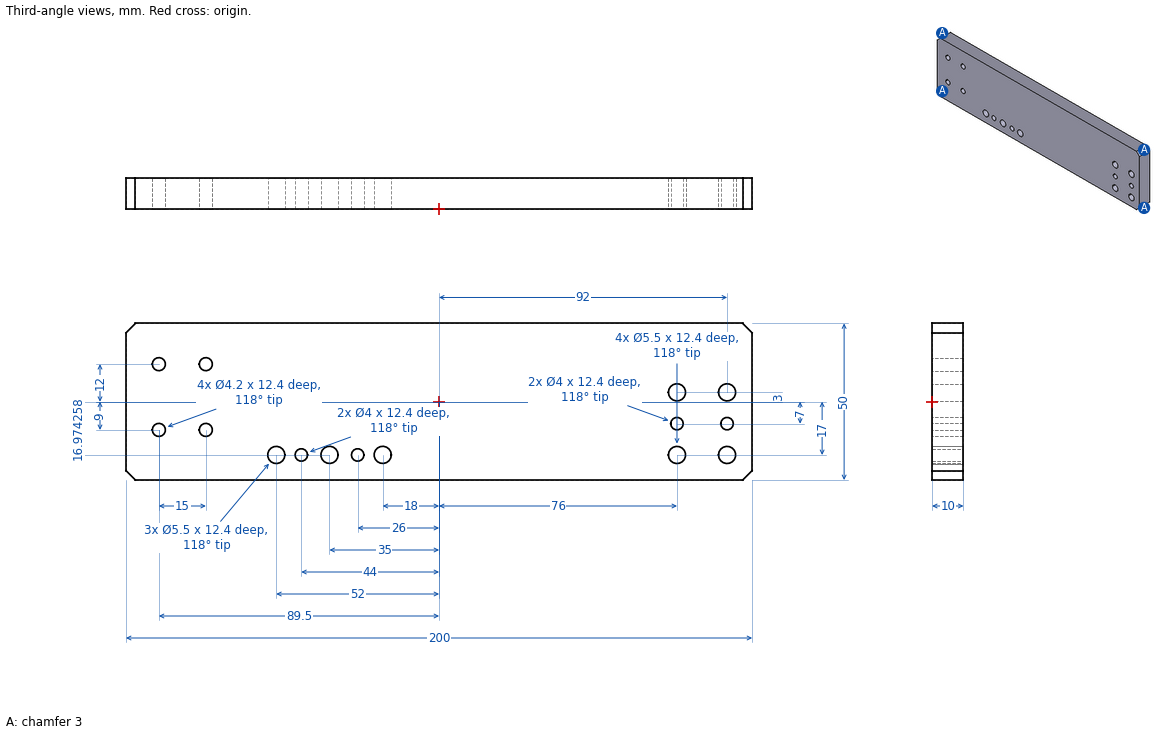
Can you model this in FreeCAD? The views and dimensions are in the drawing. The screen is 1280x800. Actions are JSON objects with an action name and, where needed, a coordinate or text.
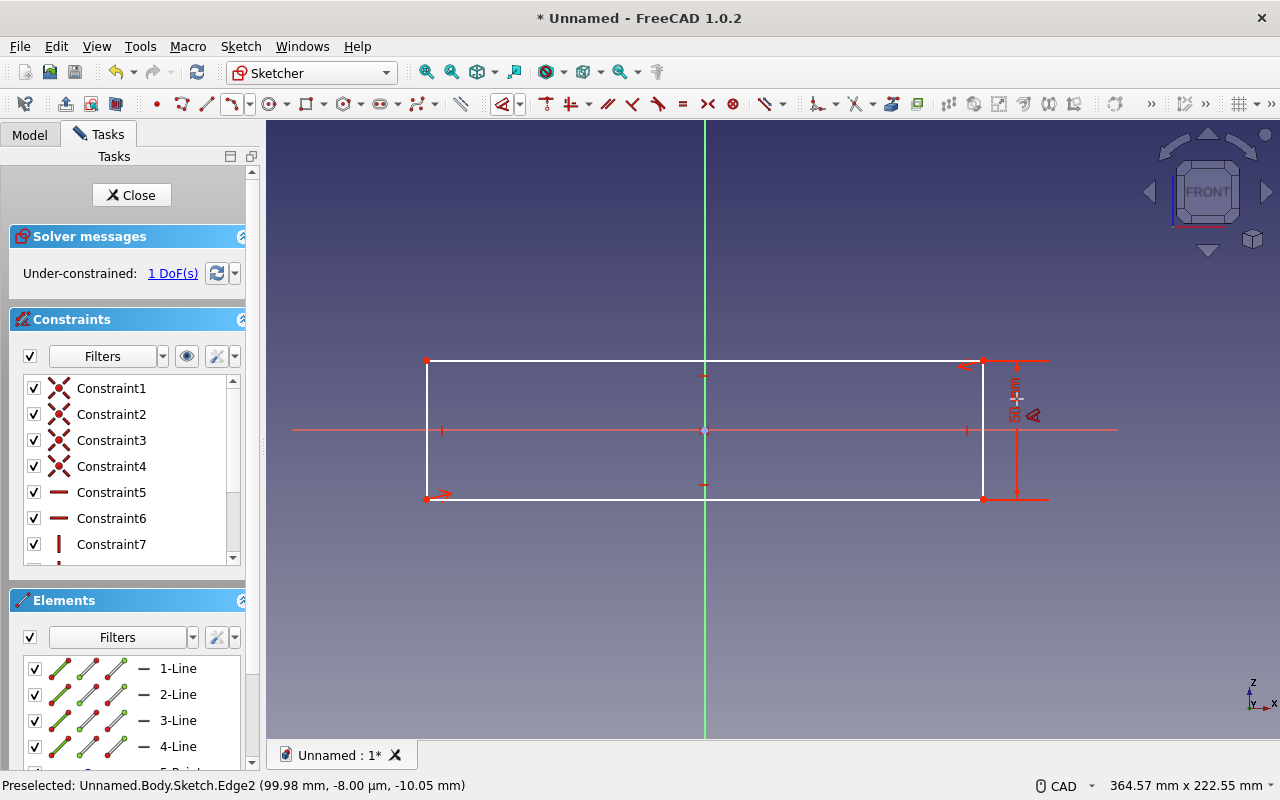
{"action": "left_click", "coordinate": [594, 500]}
{"action": "left_click", "coordinate": [577, 534]}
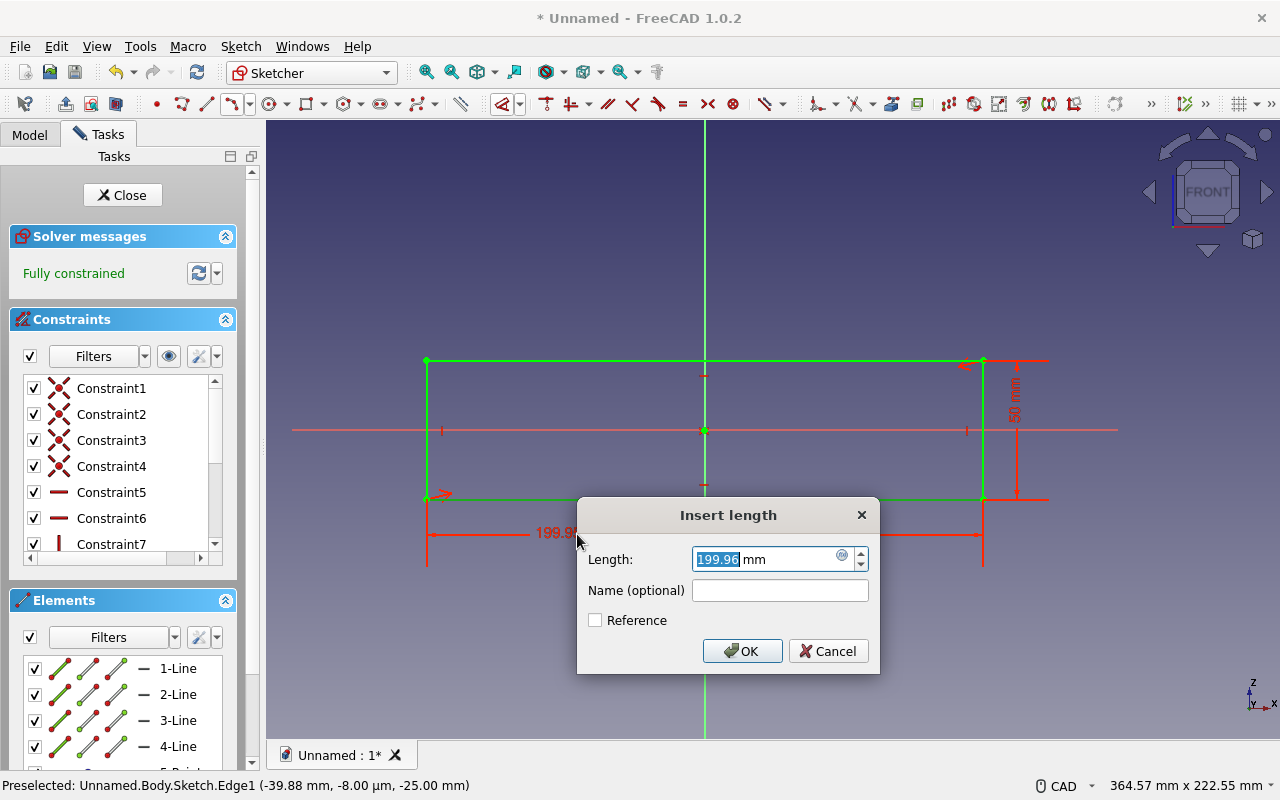
{"action": "type", "text": "200"}
{"action": "key", "text": "Return"}
{"action": "key", "text": "Escape"}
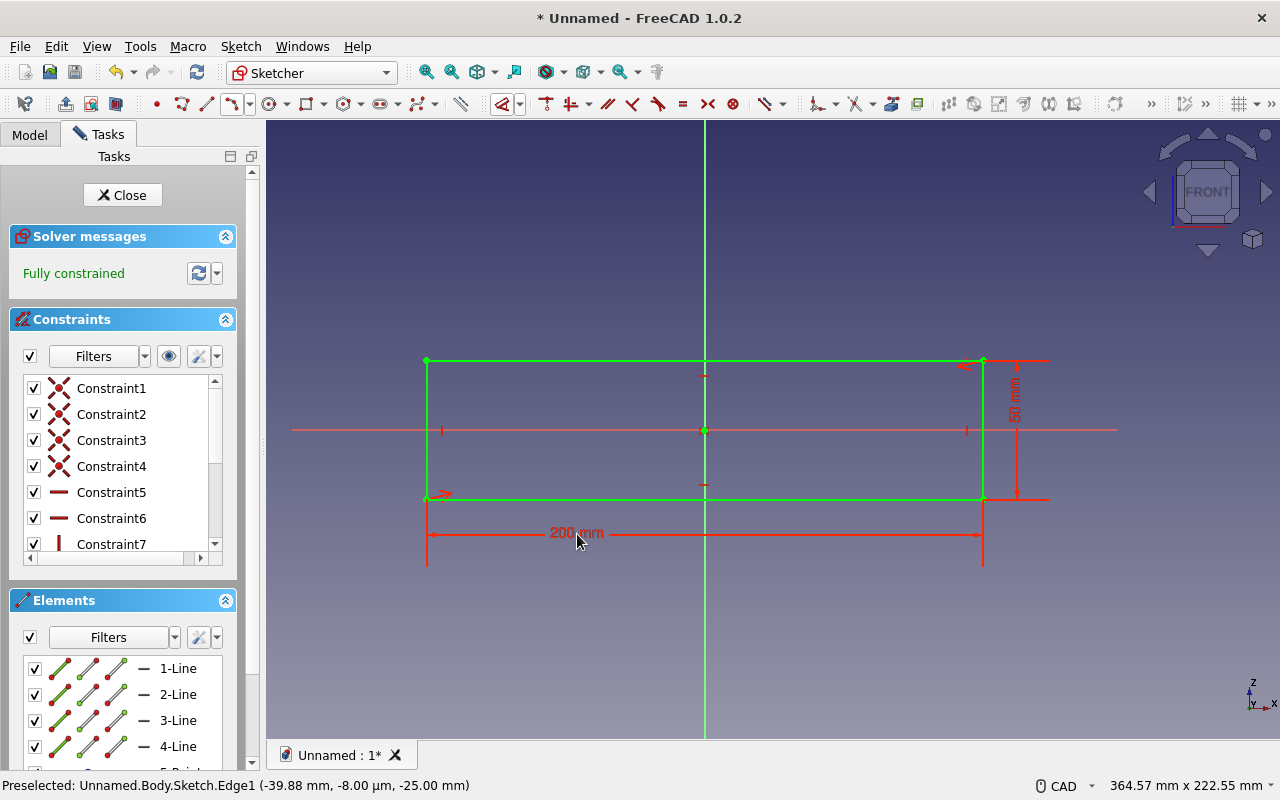
{"action": "left_click", "coordinate": [123, 195]}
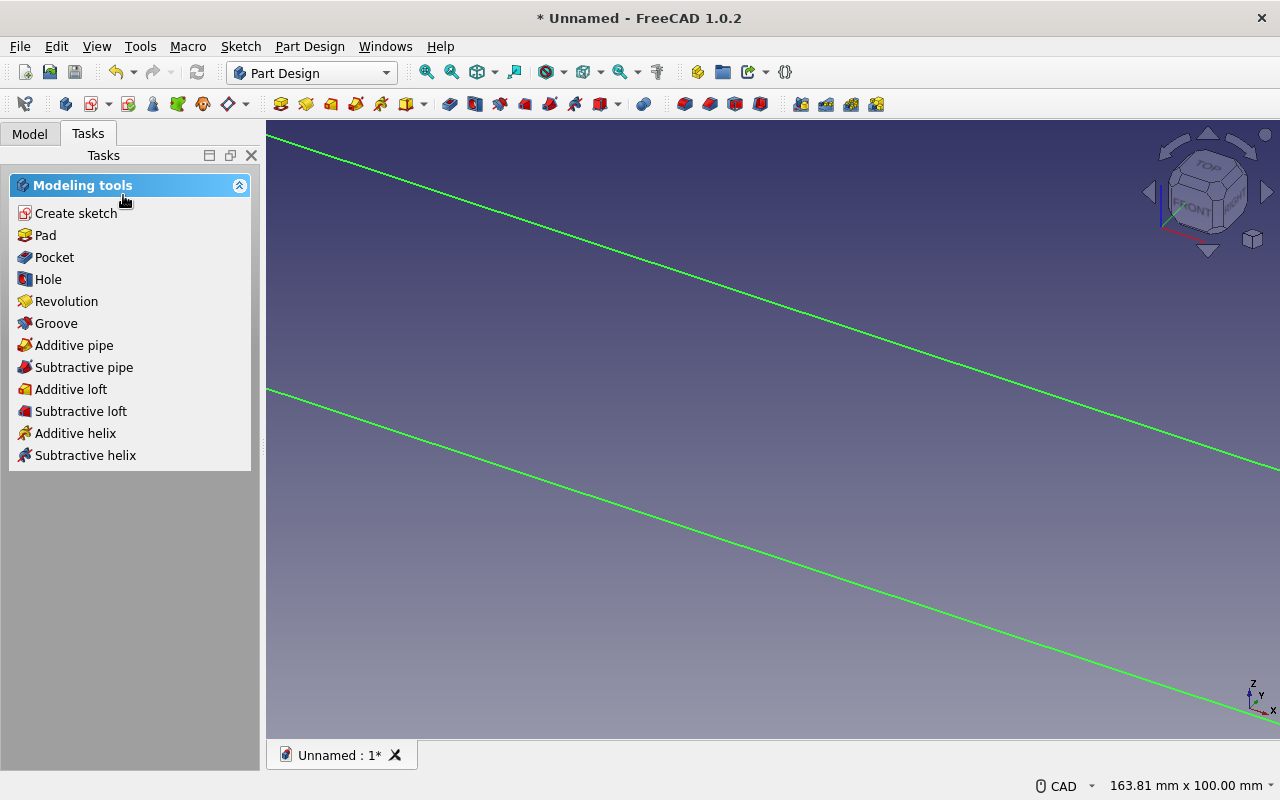
{"action": "left_click", "coordinate": [281, 104]}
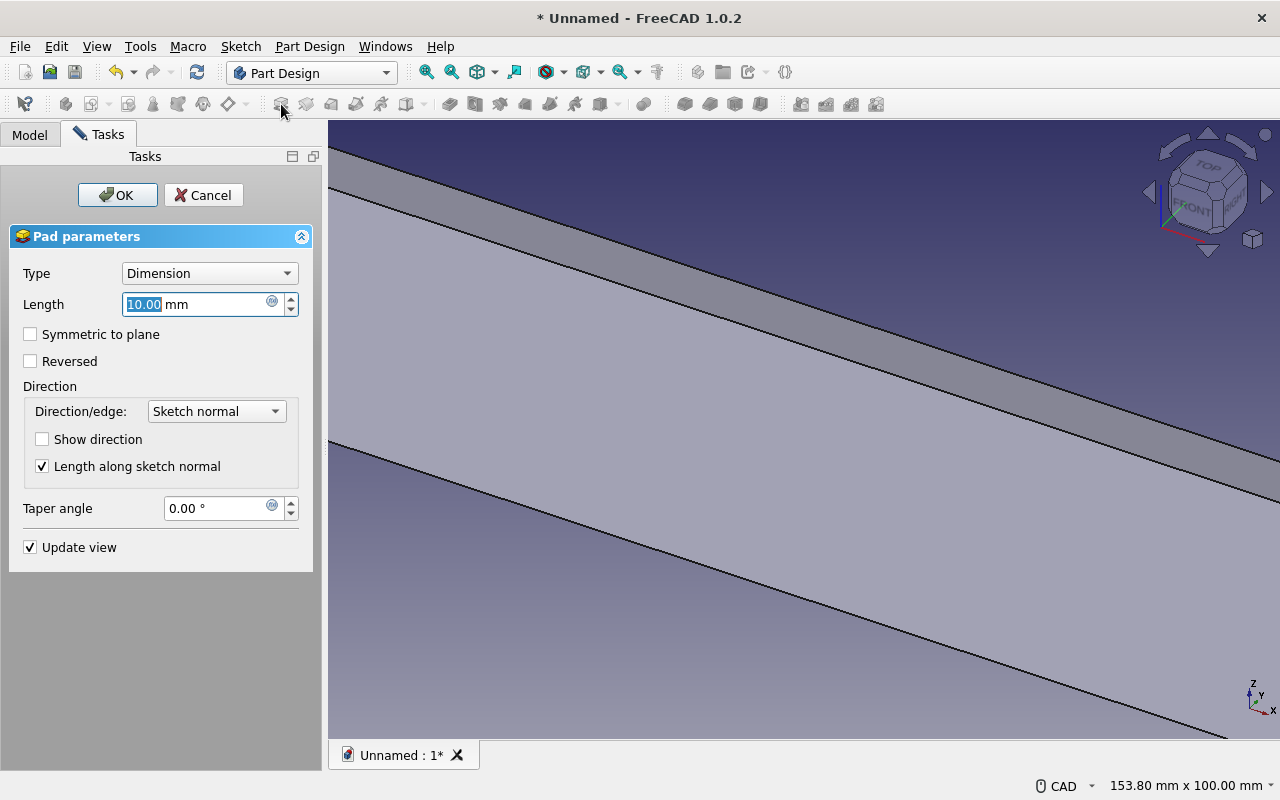
{"action": "type", "text": "10"}
{"action": "key", "text": "Tab"}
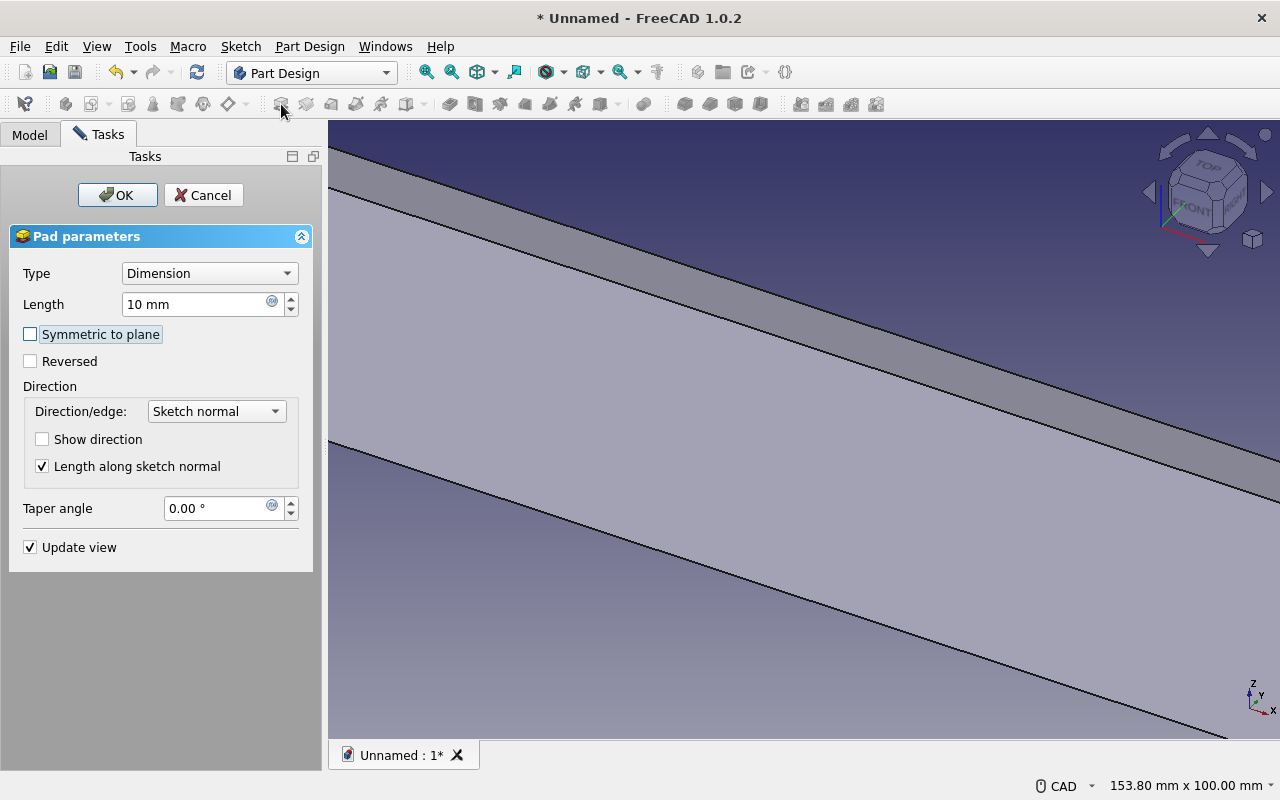
{"action": "left_click", "coordinate": [31, 361]}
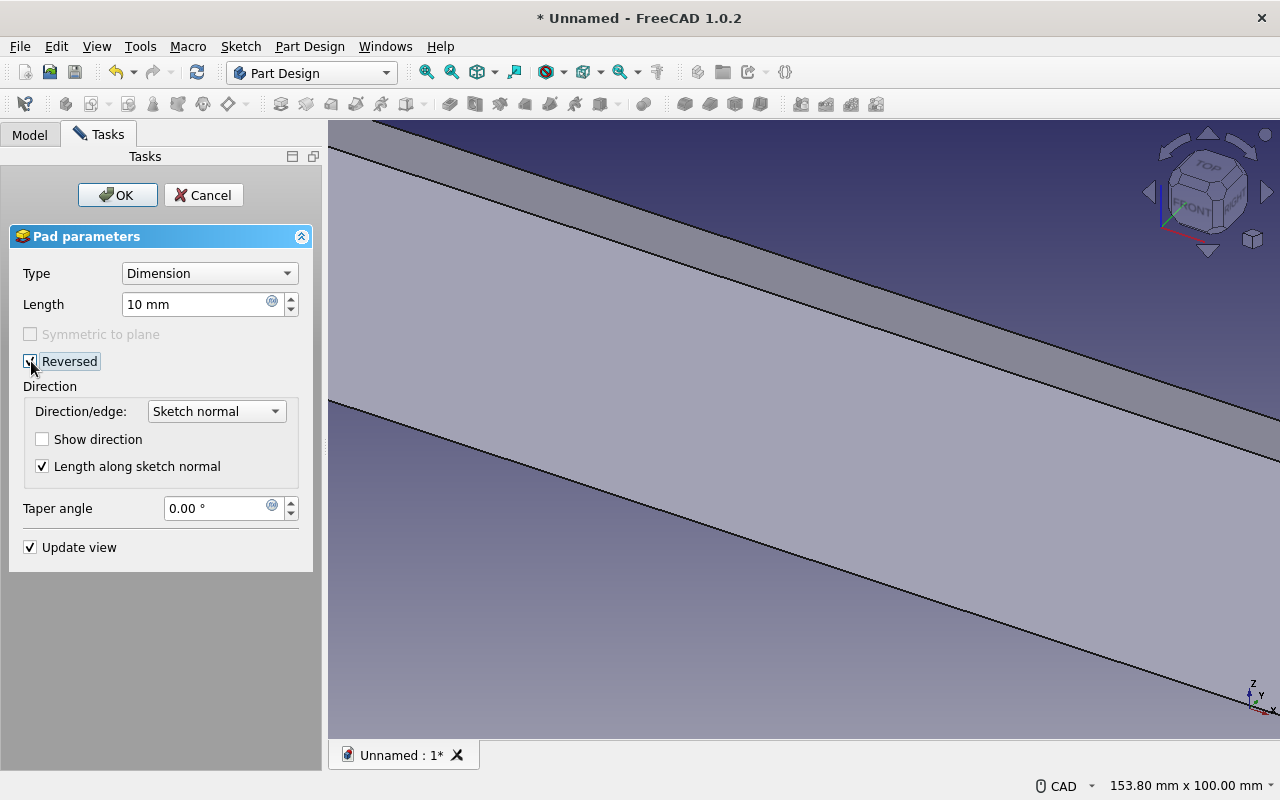
{"action": "left_click", "coordinate": [118, 195]}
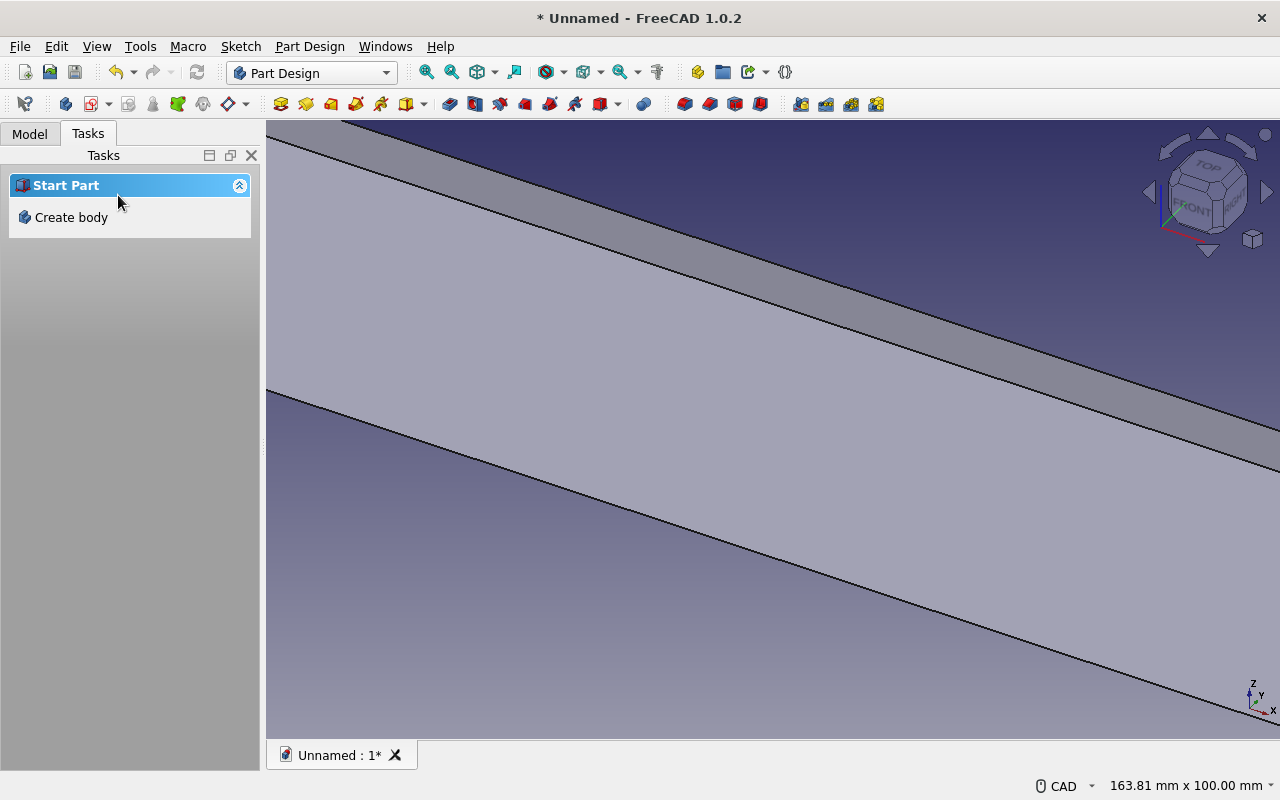
{"action": "key", "text": "v f"}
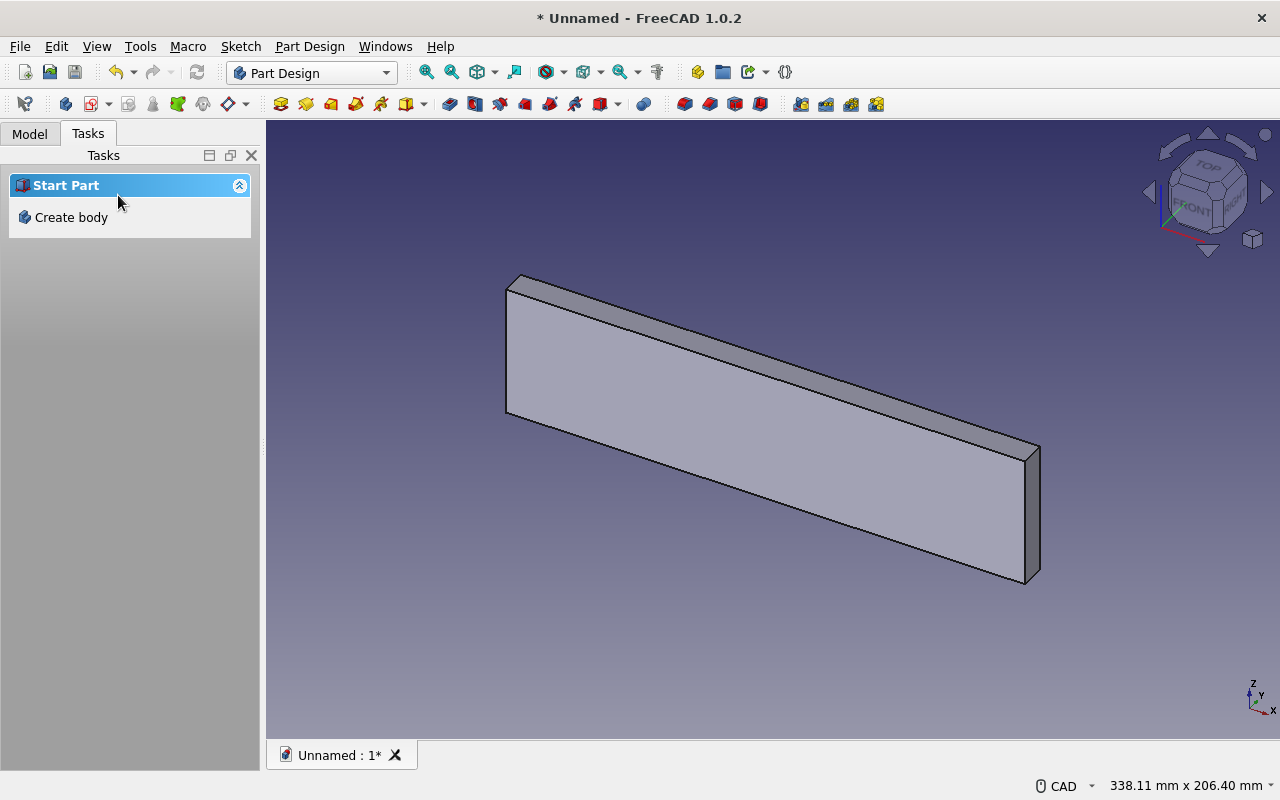
{"action": "left_click", "coordinate": [1033, 453]}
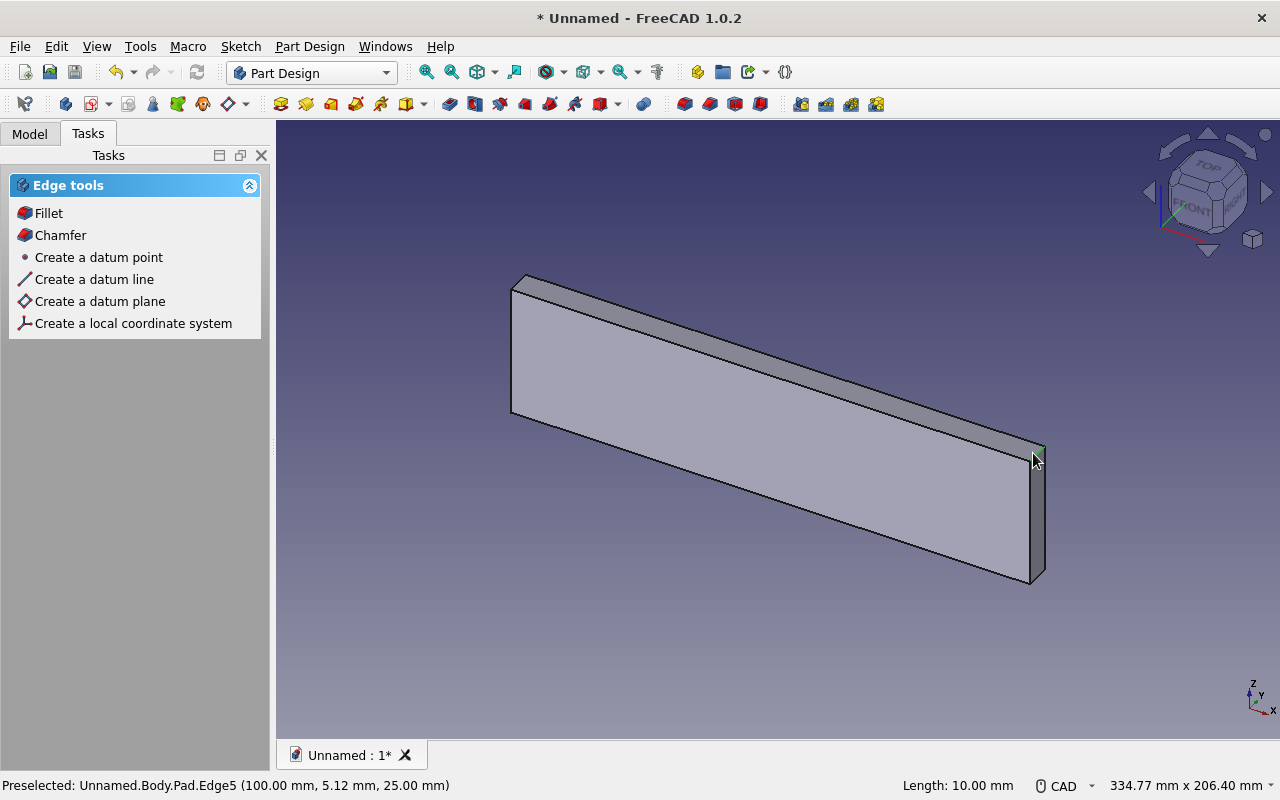
{"action": "key", "text": "0"}